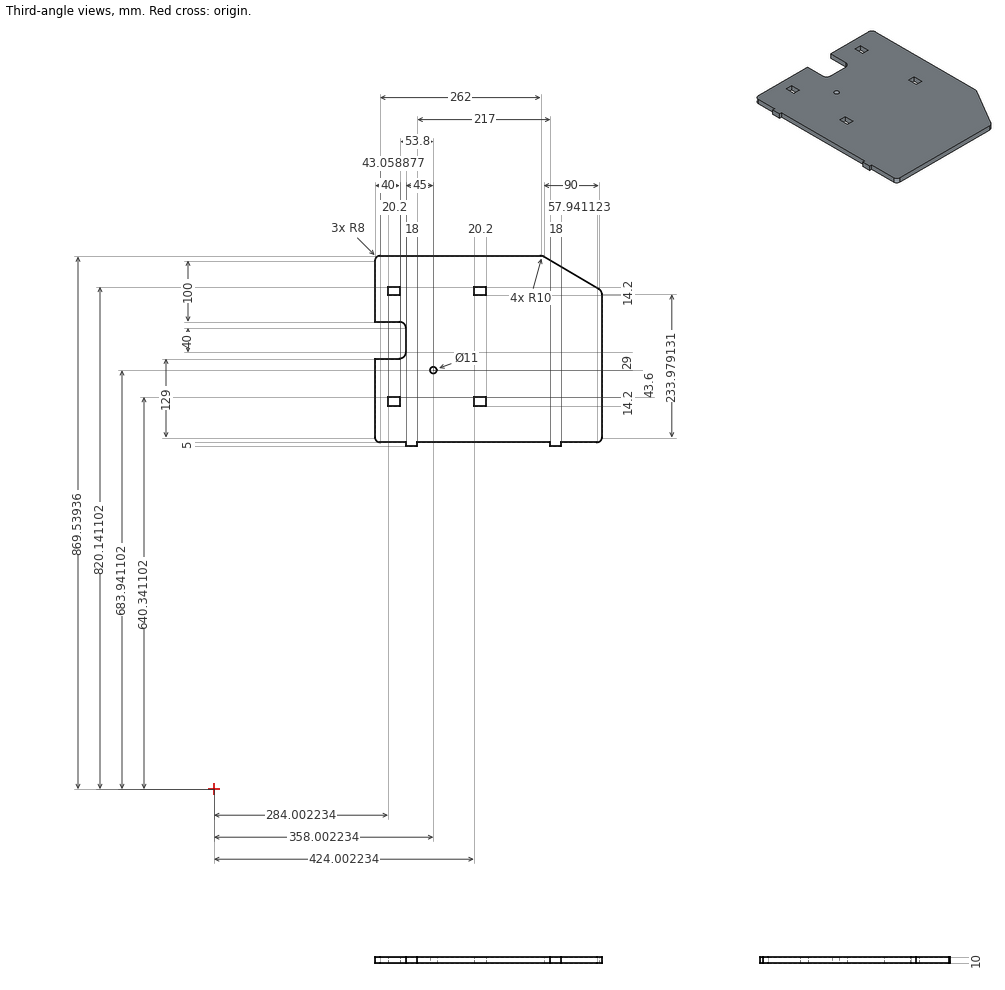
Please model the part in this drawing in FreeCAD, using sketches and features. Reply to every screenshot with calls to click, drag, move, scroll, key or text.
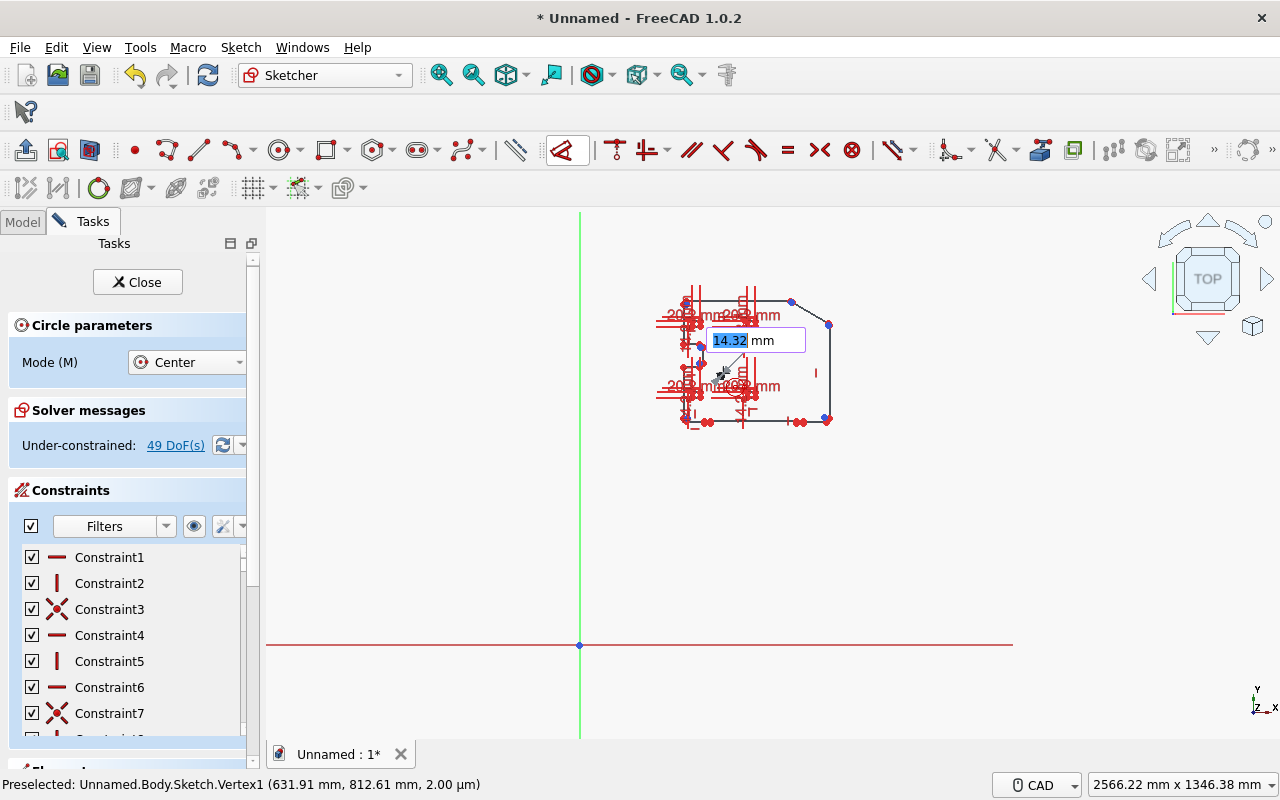
text(11)
key(Return)
key(Escape)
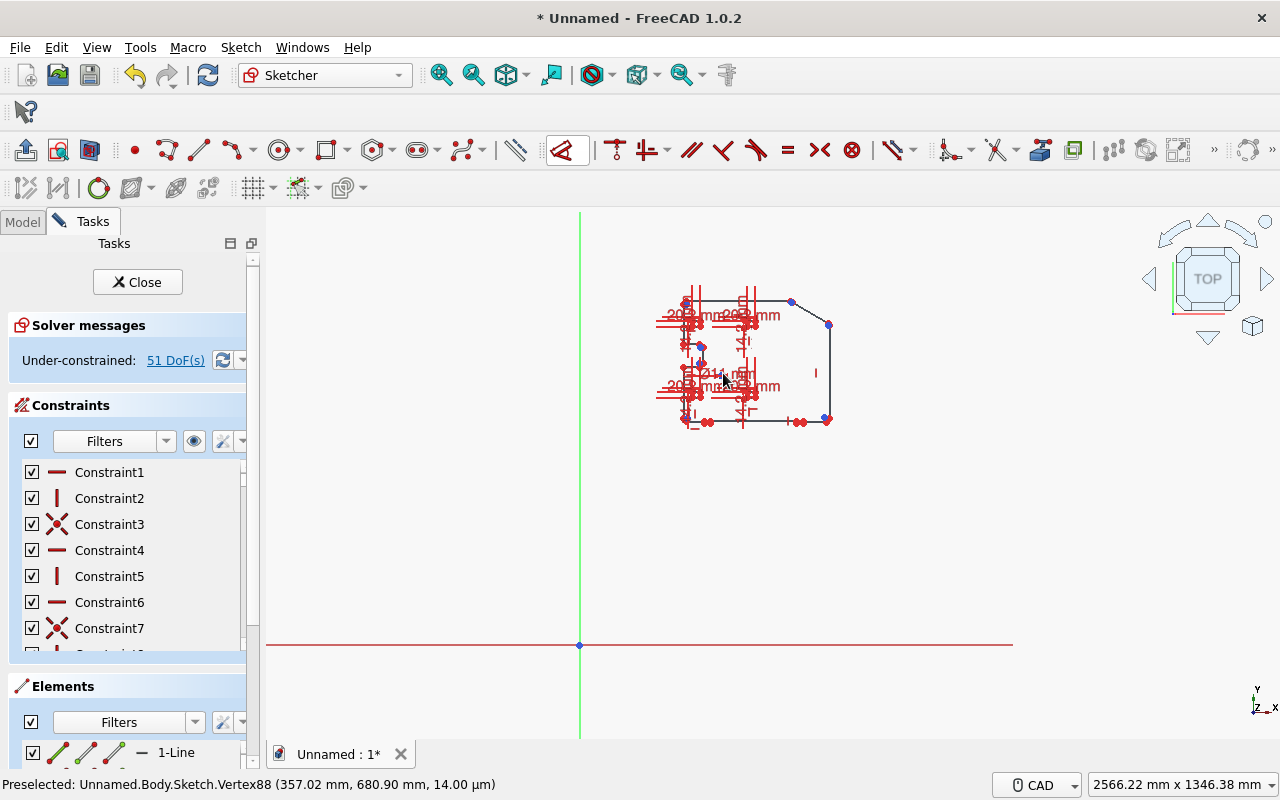
click(759, 301)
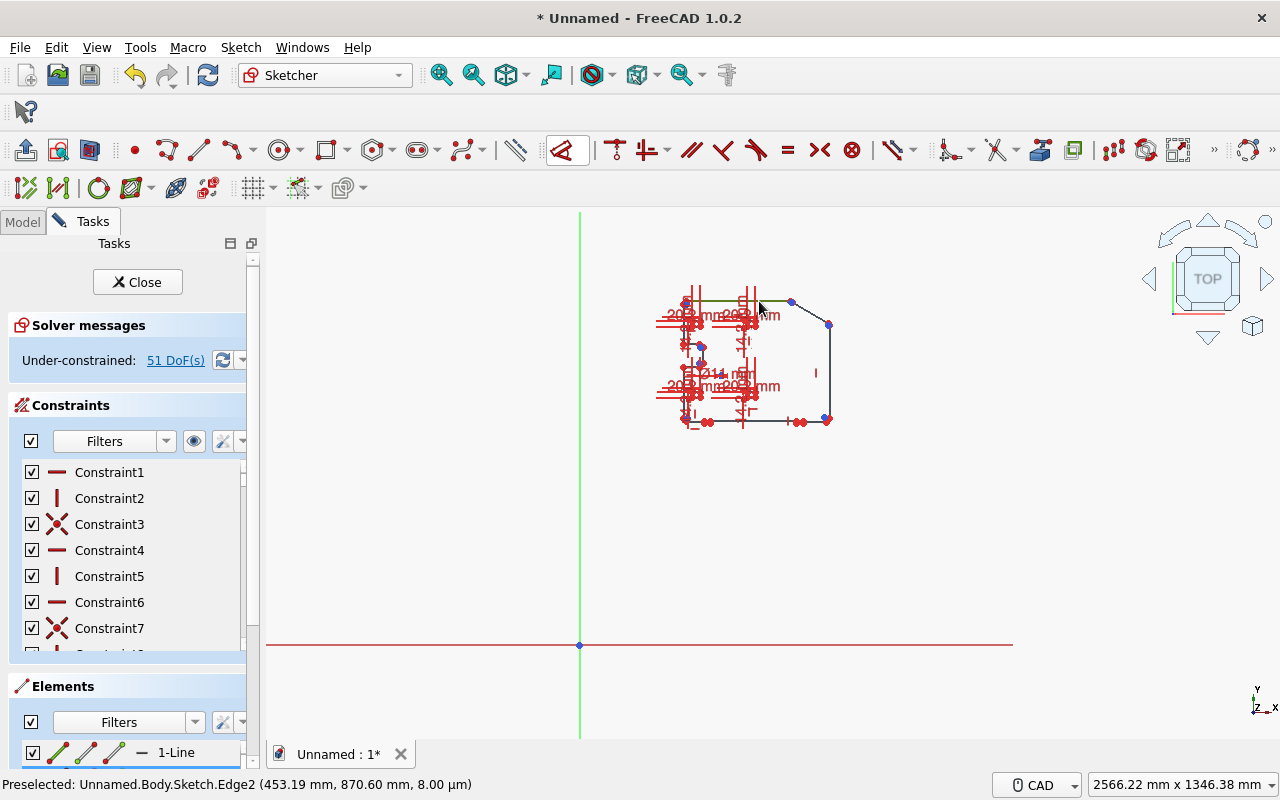
scroll(792, 301, up, 12)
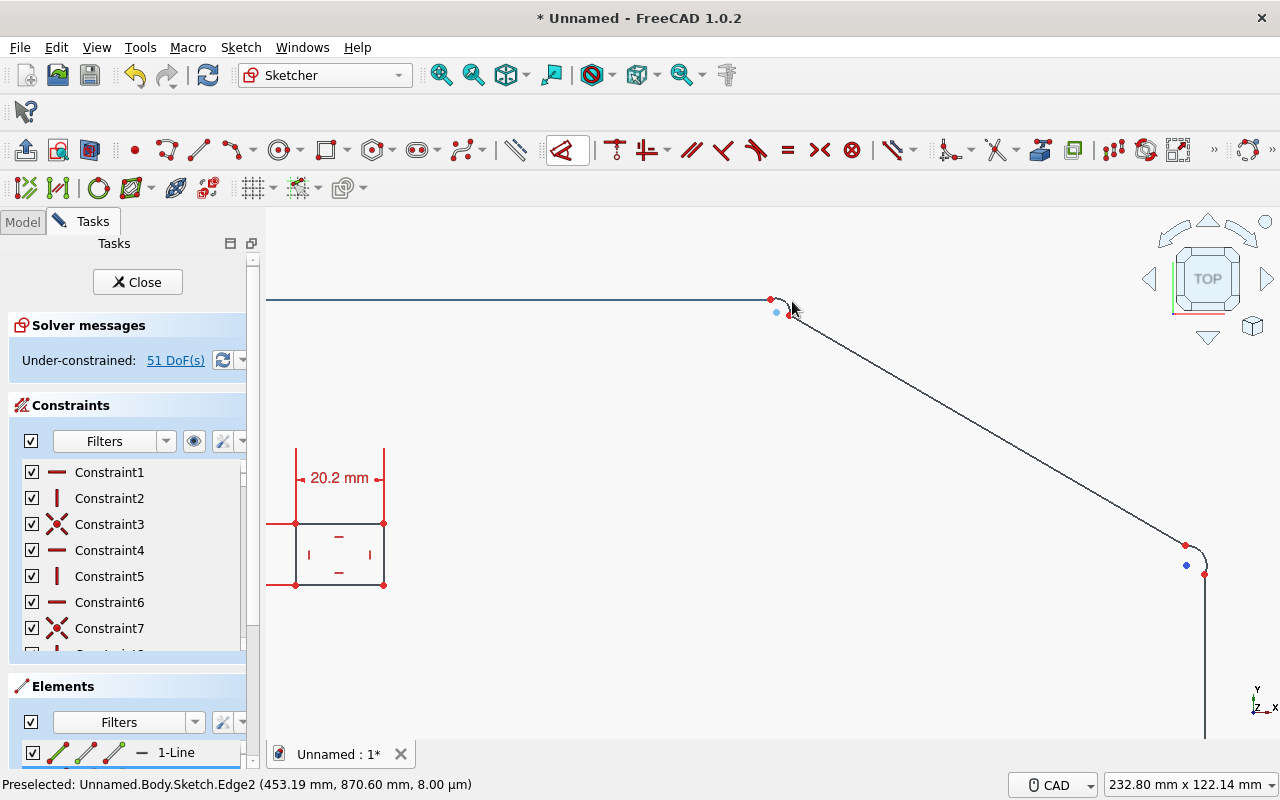
click(785, 301)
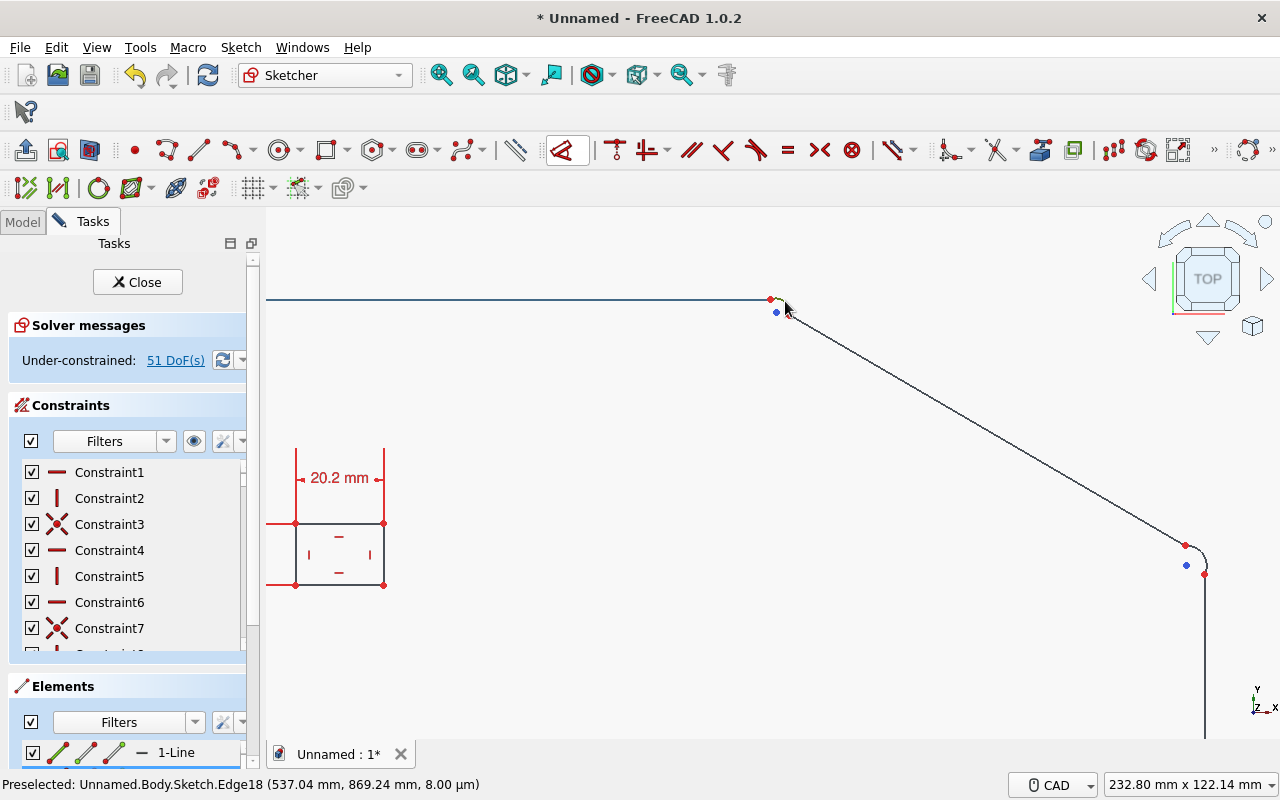
click(756, 150)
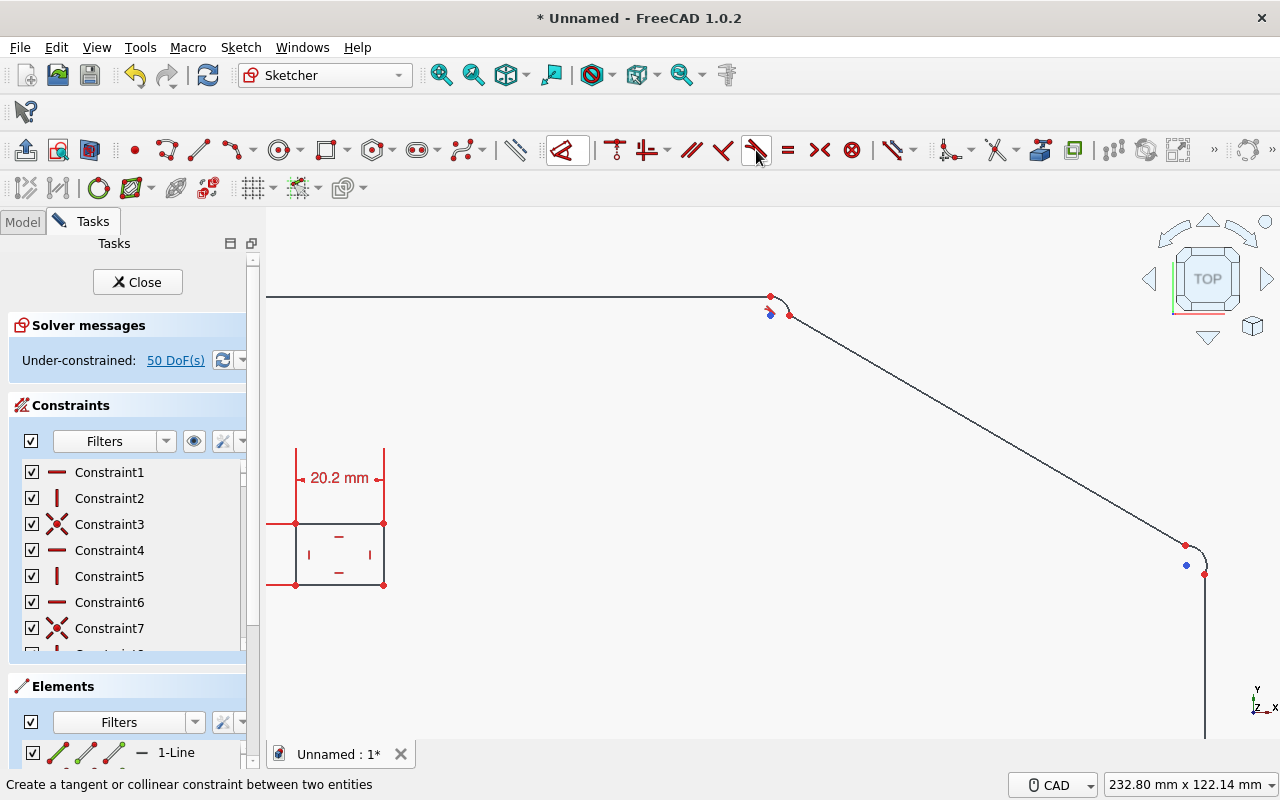
scroll(792, 301, down, 12)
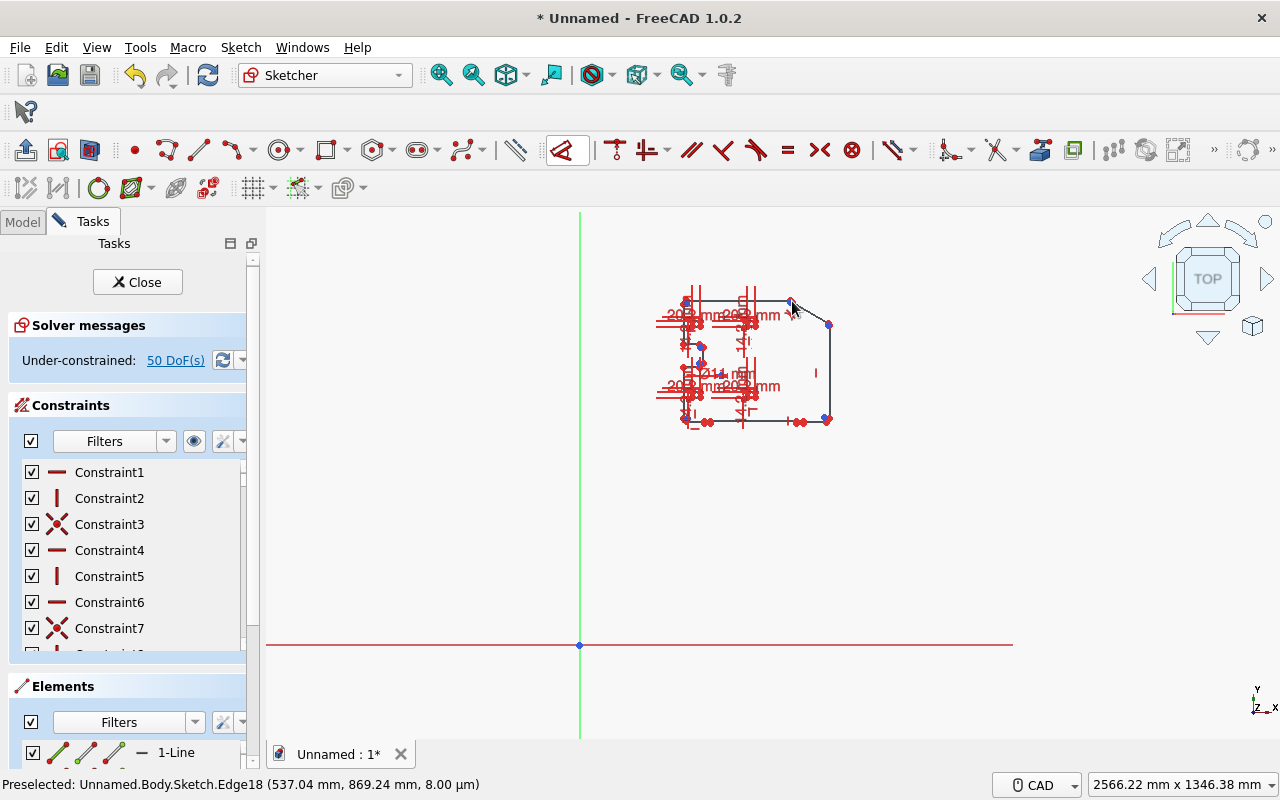
click(759, 301)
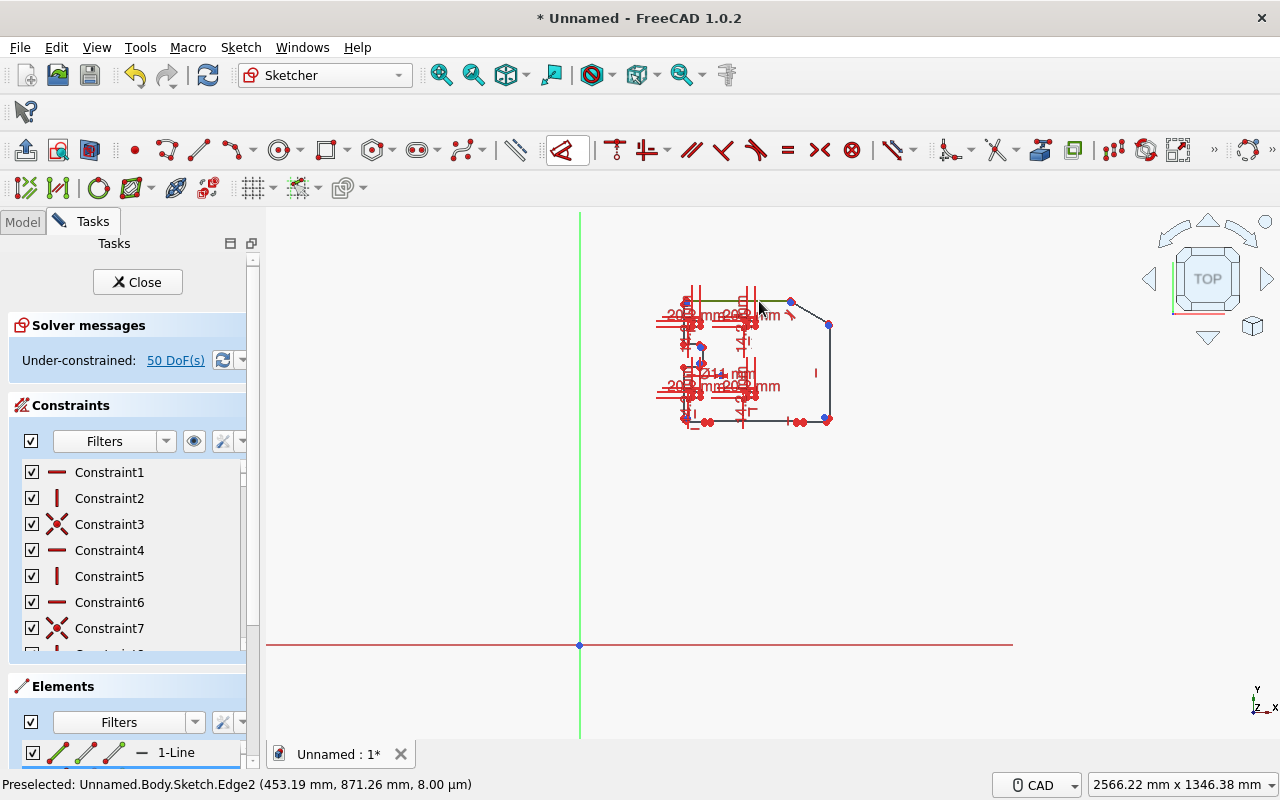
scroll(685, 302, up, 9)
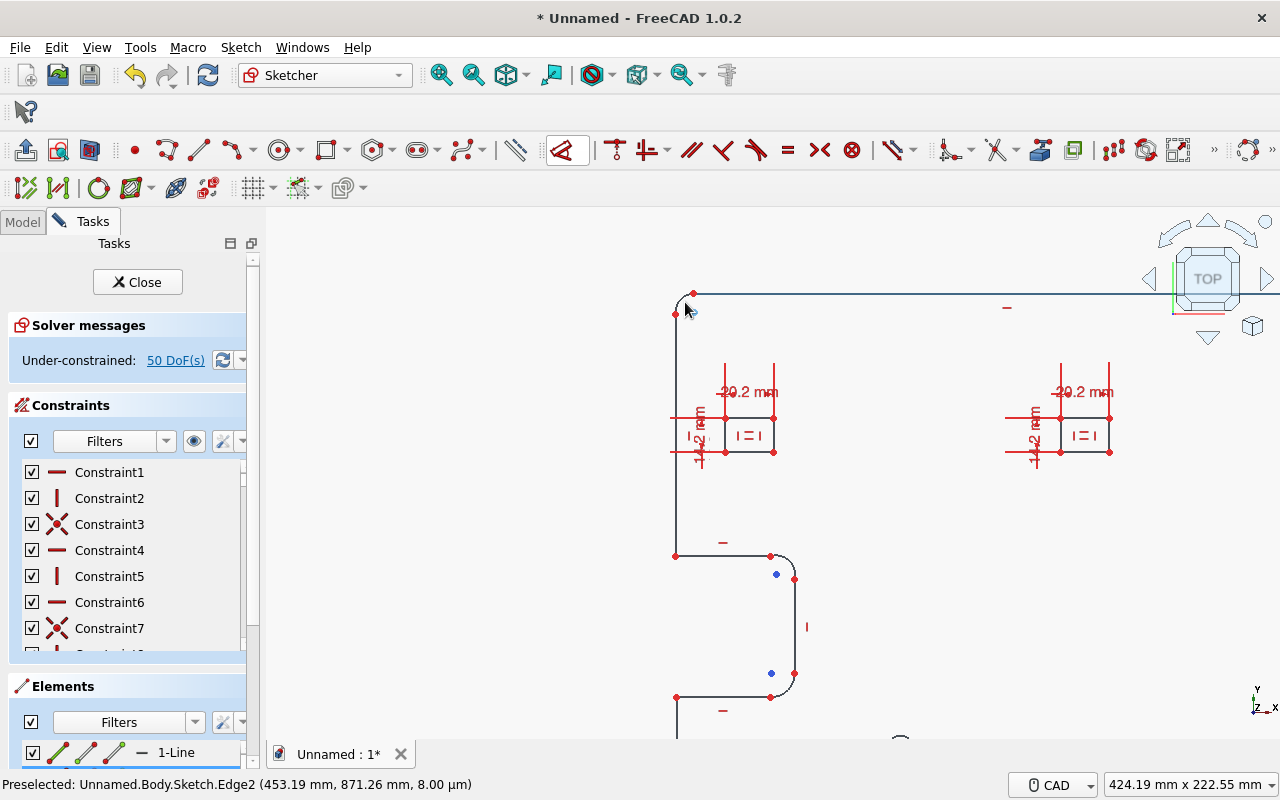
click(680, 300)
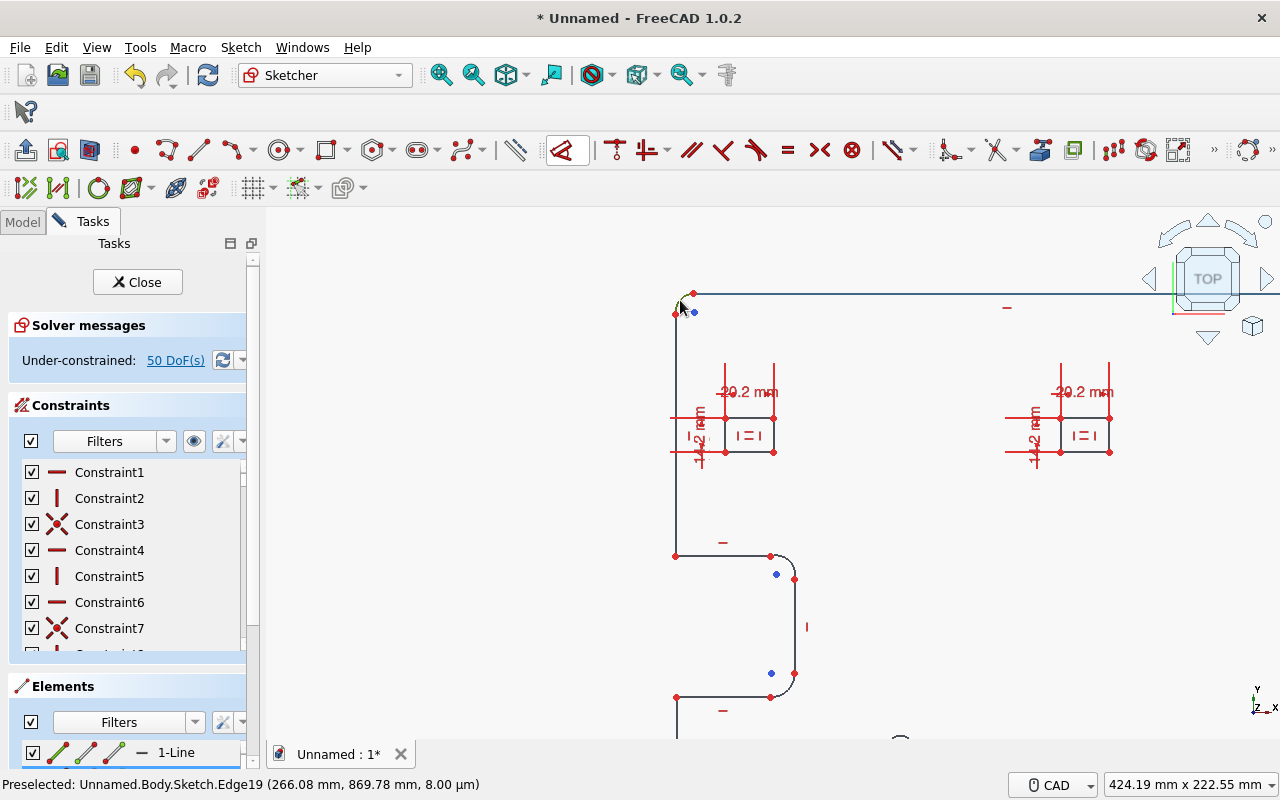
click(756, 150)